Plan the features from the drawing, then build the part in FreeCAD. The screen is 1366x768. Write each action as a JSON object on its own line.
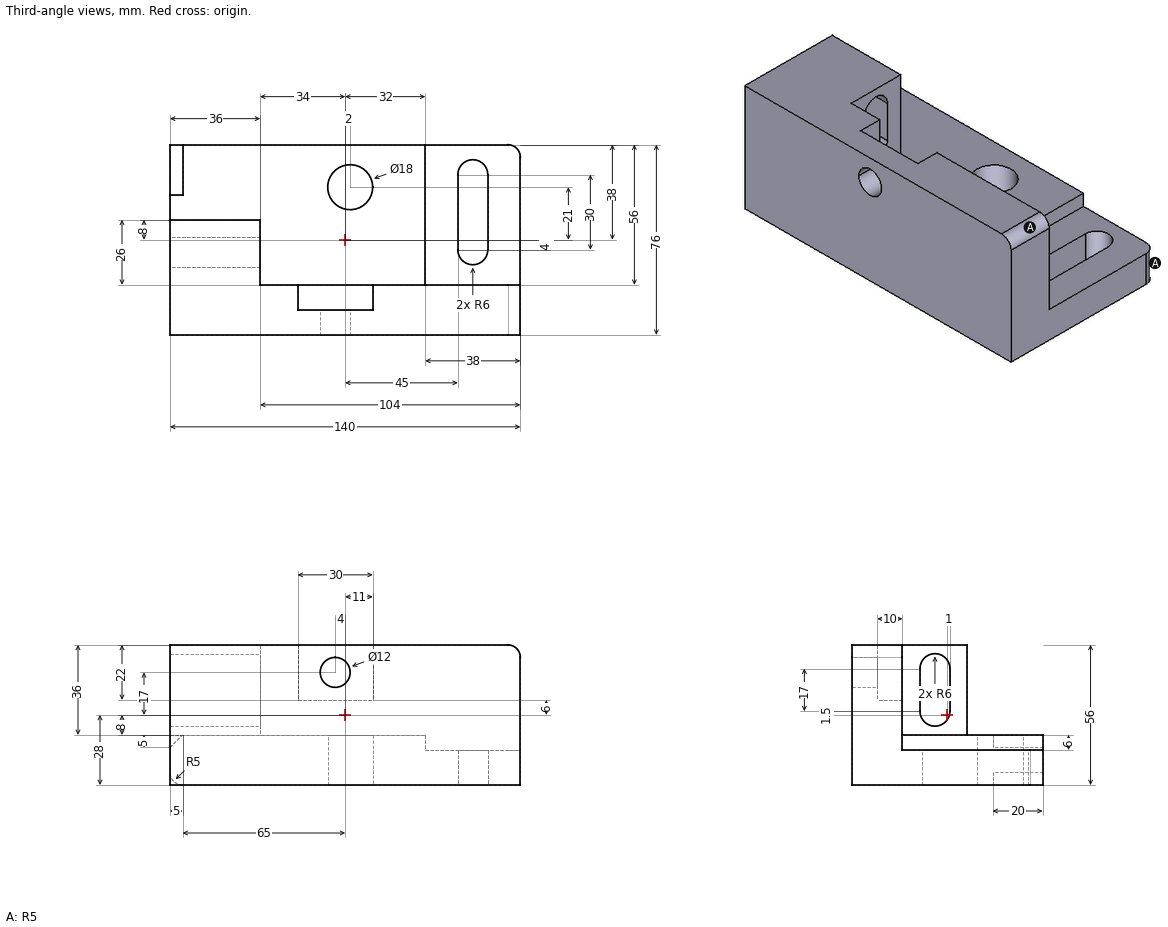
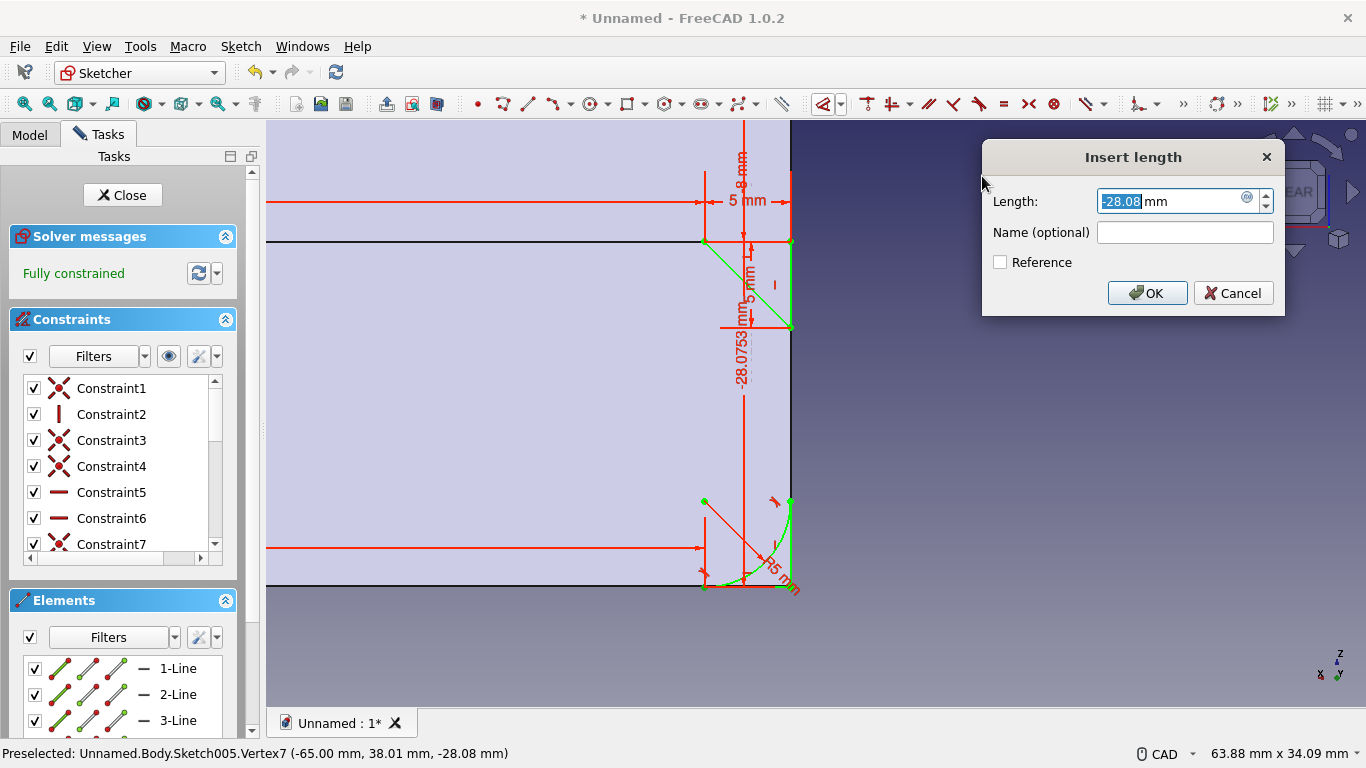
{"action": "type", "text": "-28"}
{"action": "key", "text": "Return"}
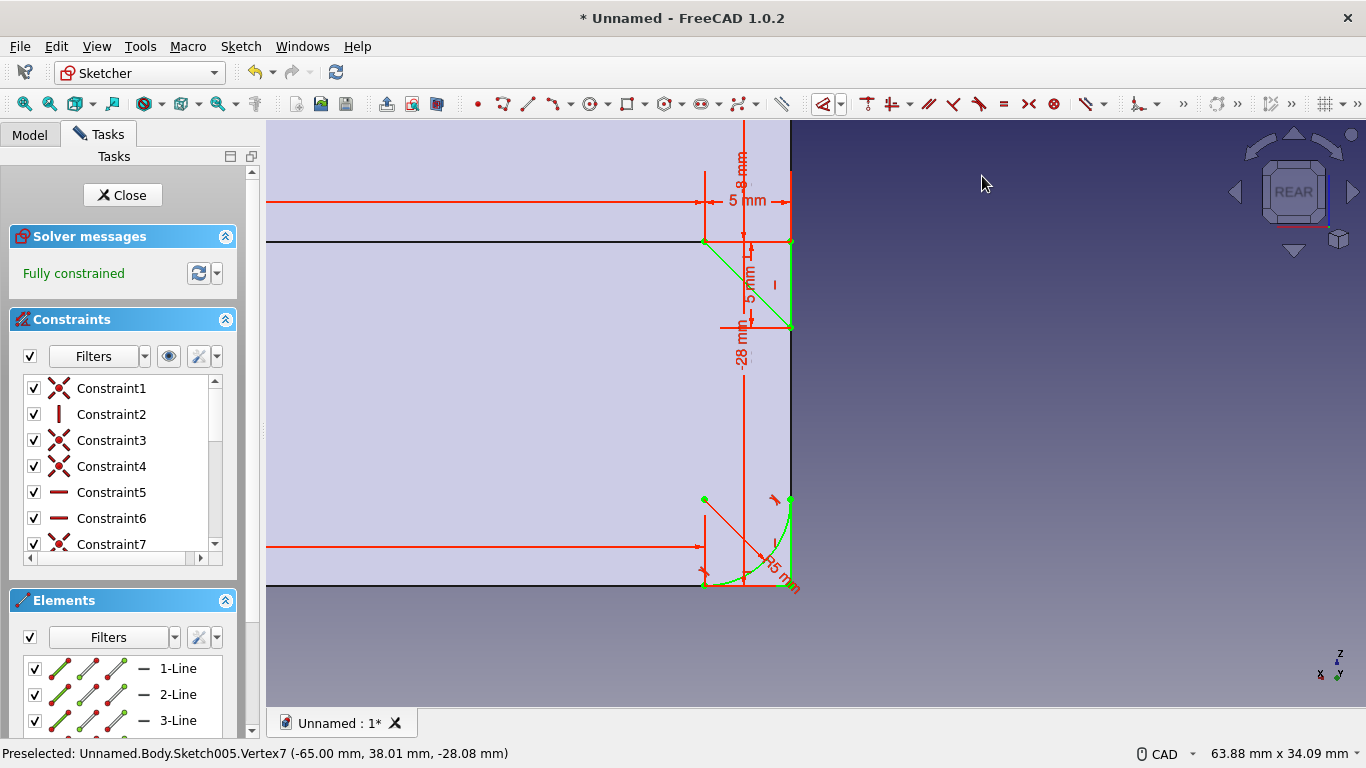
{"action": "left_click", "coordinate": [123, 195]}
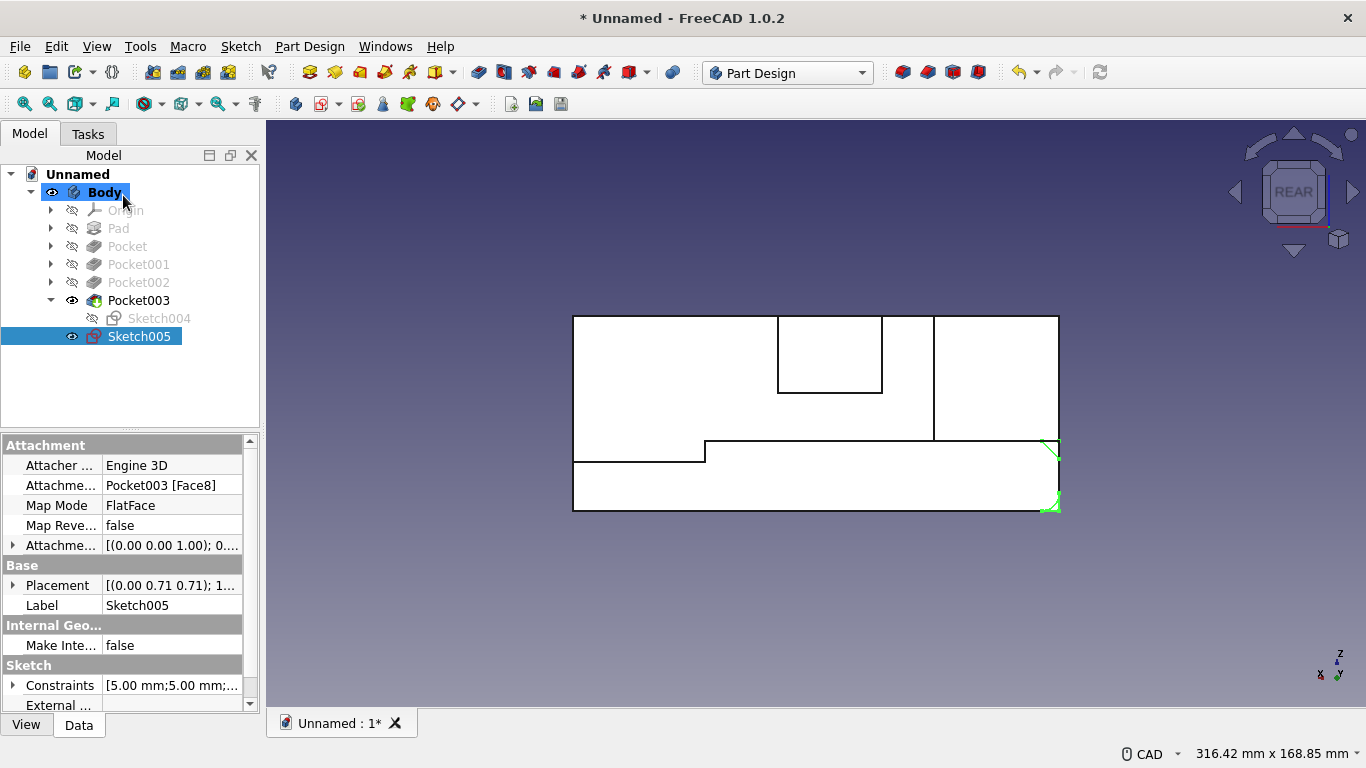
{"action": "left_click", "coordinate": [479, 72]}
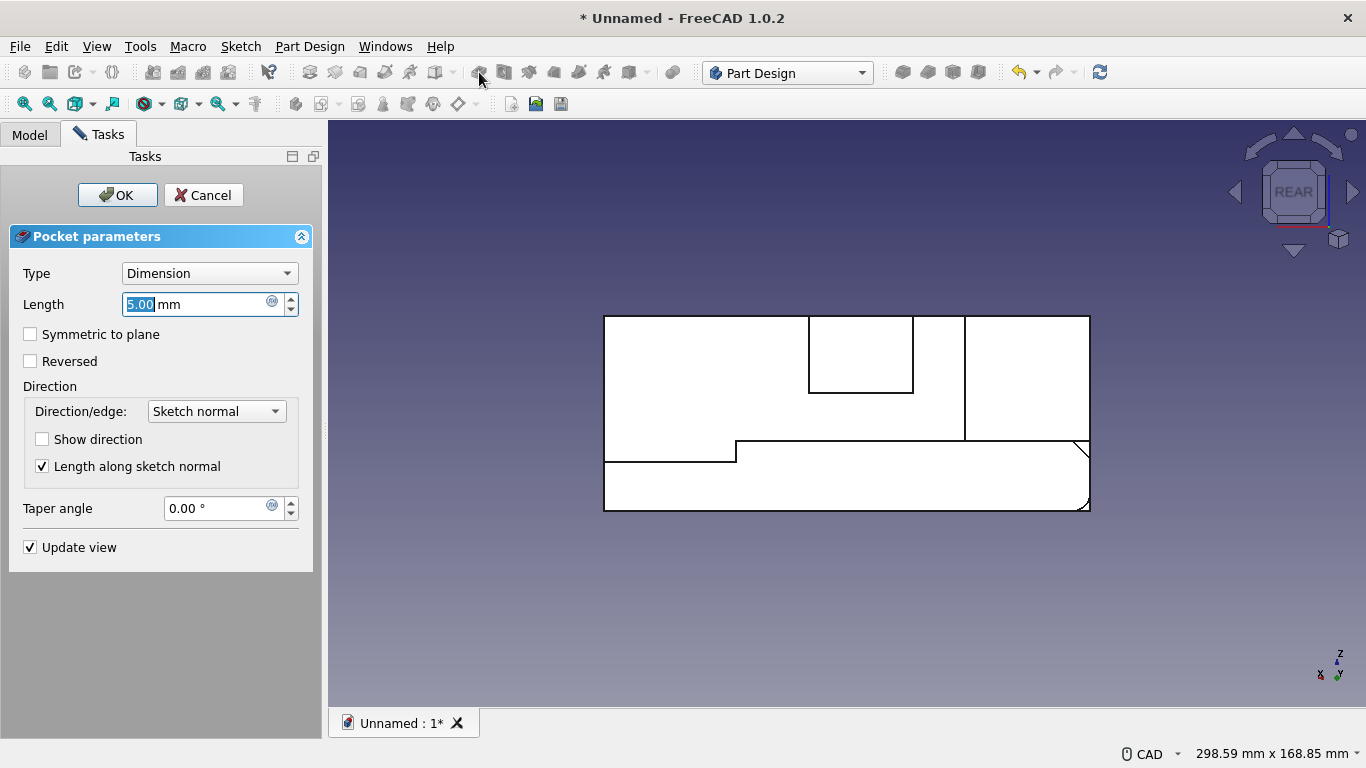
{"action": "type", "text": "20"}
{"action": "key", "text": "Tab"}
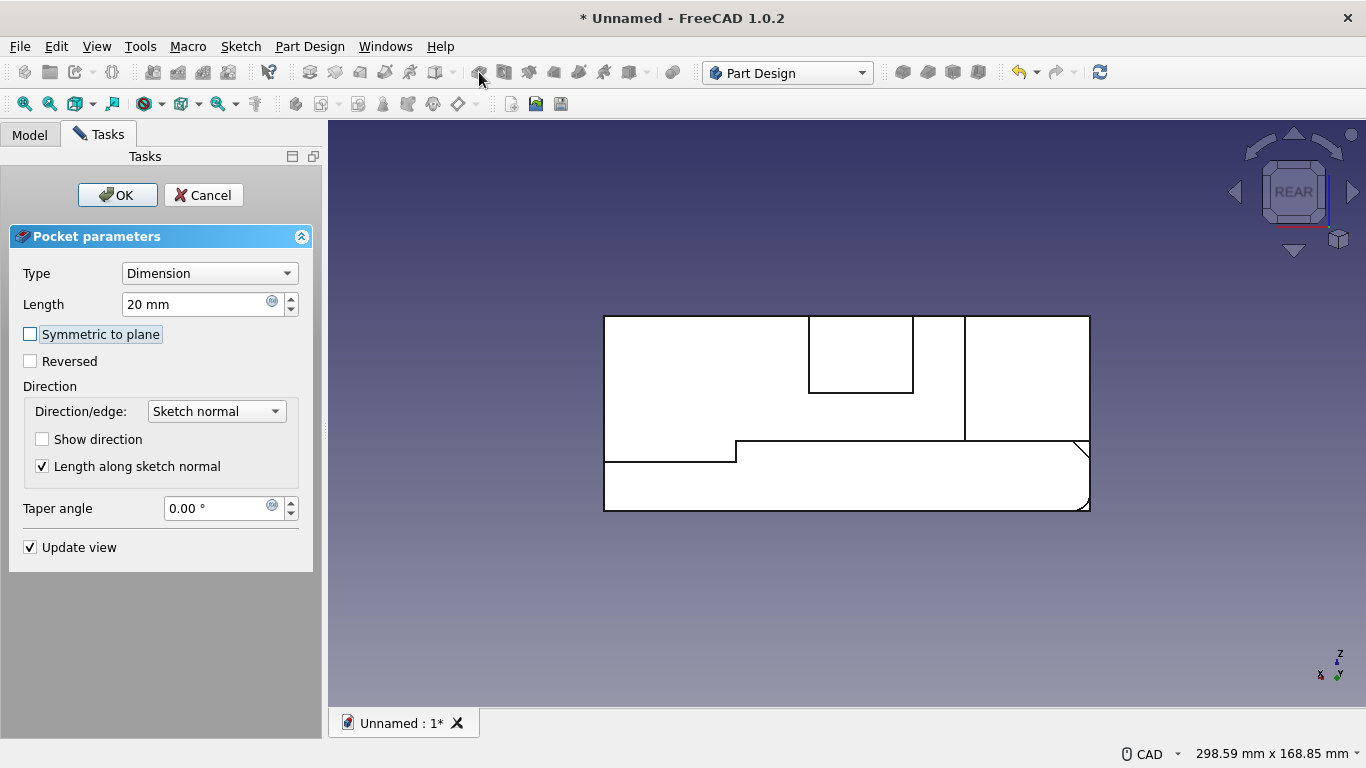
{"action": "left_click", "coordinate": [118, 195]}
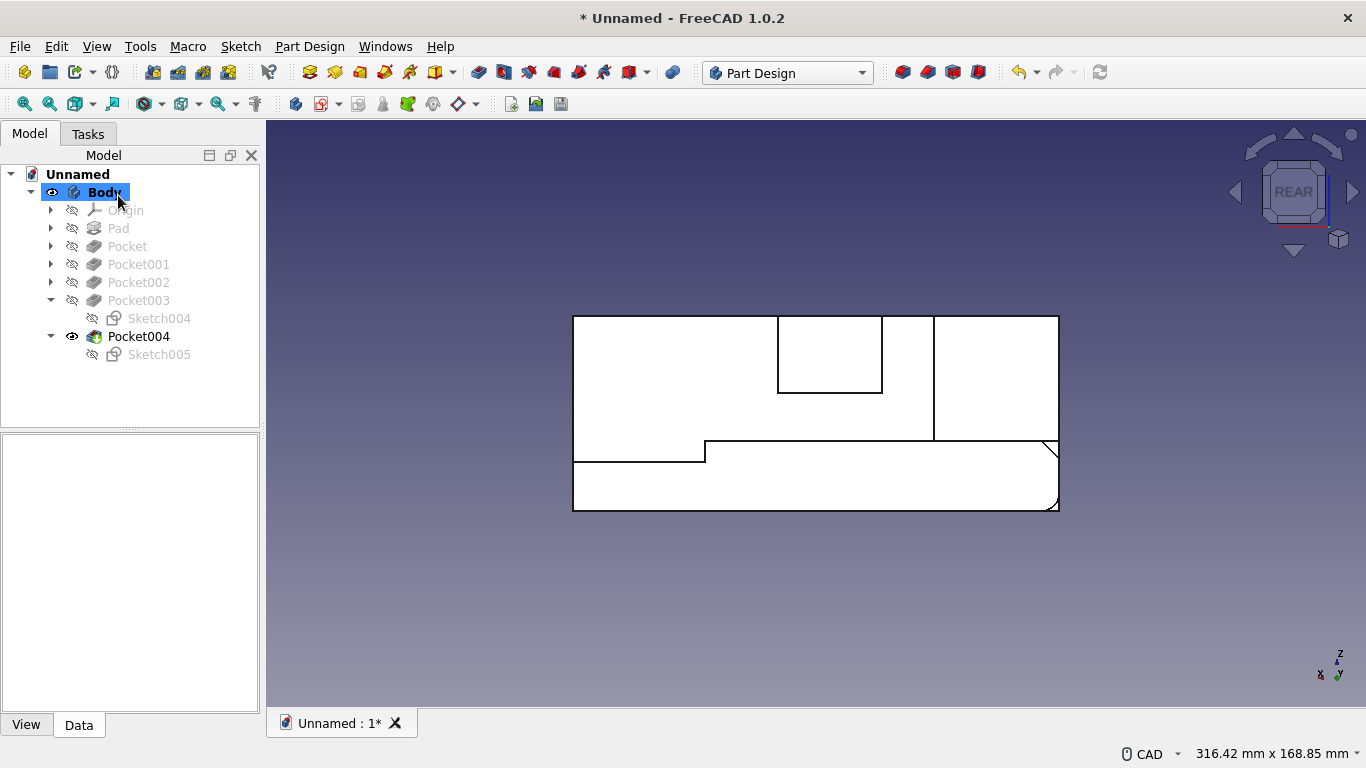
{"action": "left_click", "coordinate": [25, 104]}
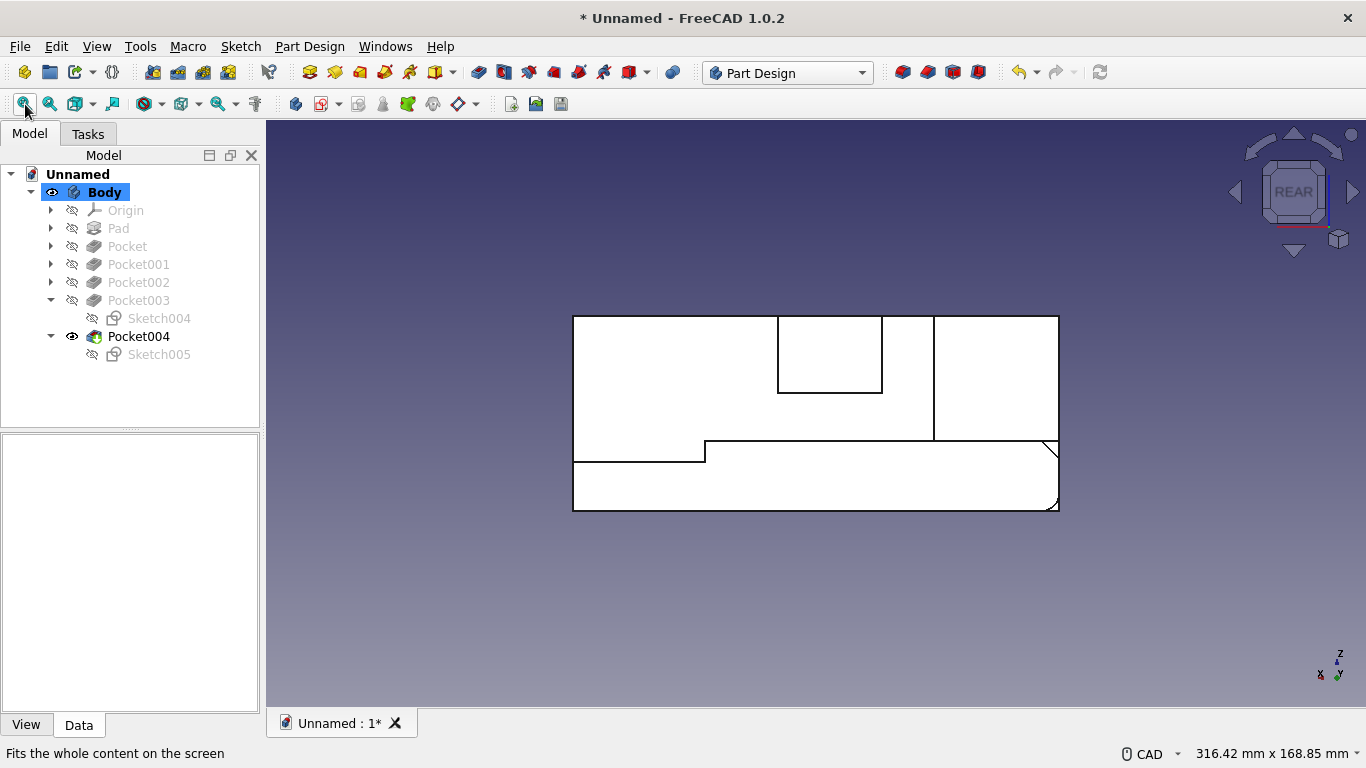
{"action": "key", "text": "0"}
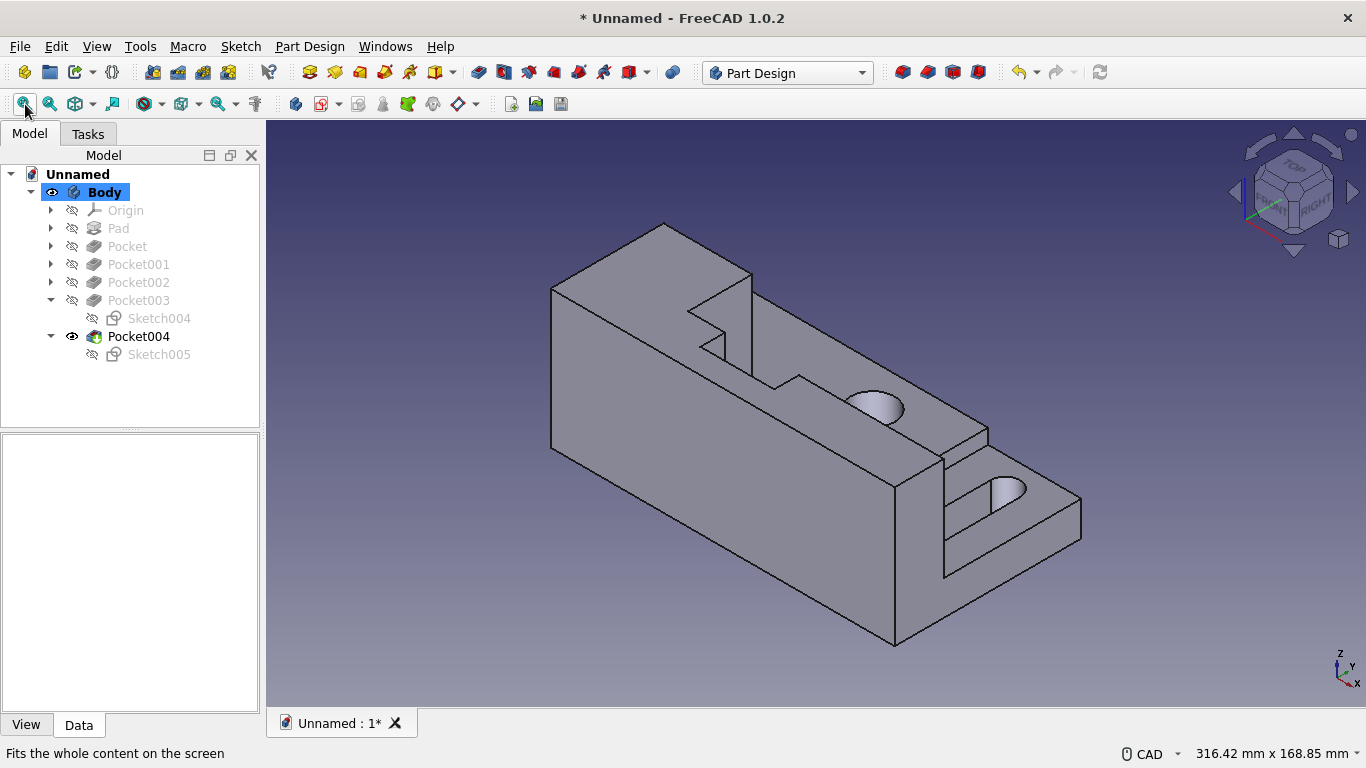
{"action": "left_click", "coordinate": [729, 323]}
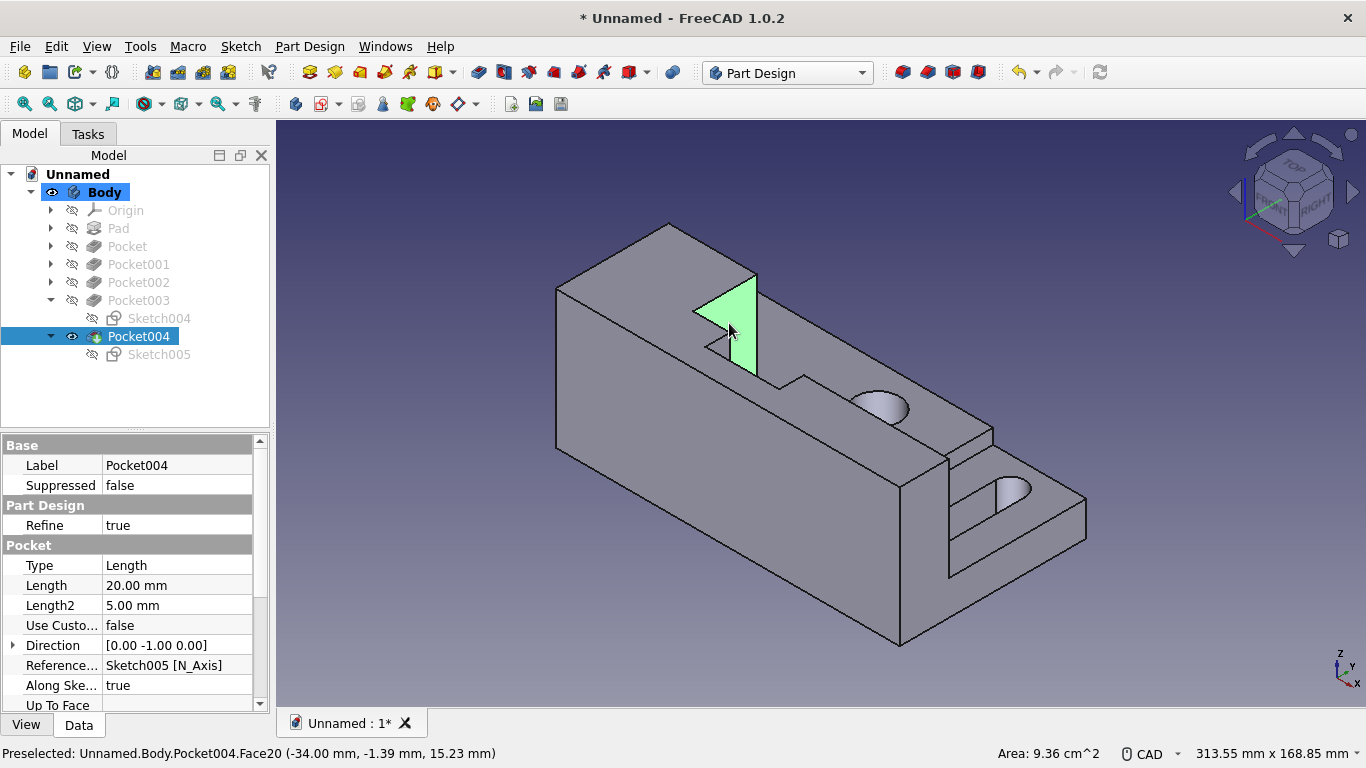
{"action": "left_click", "coordinate": [320, 104]}